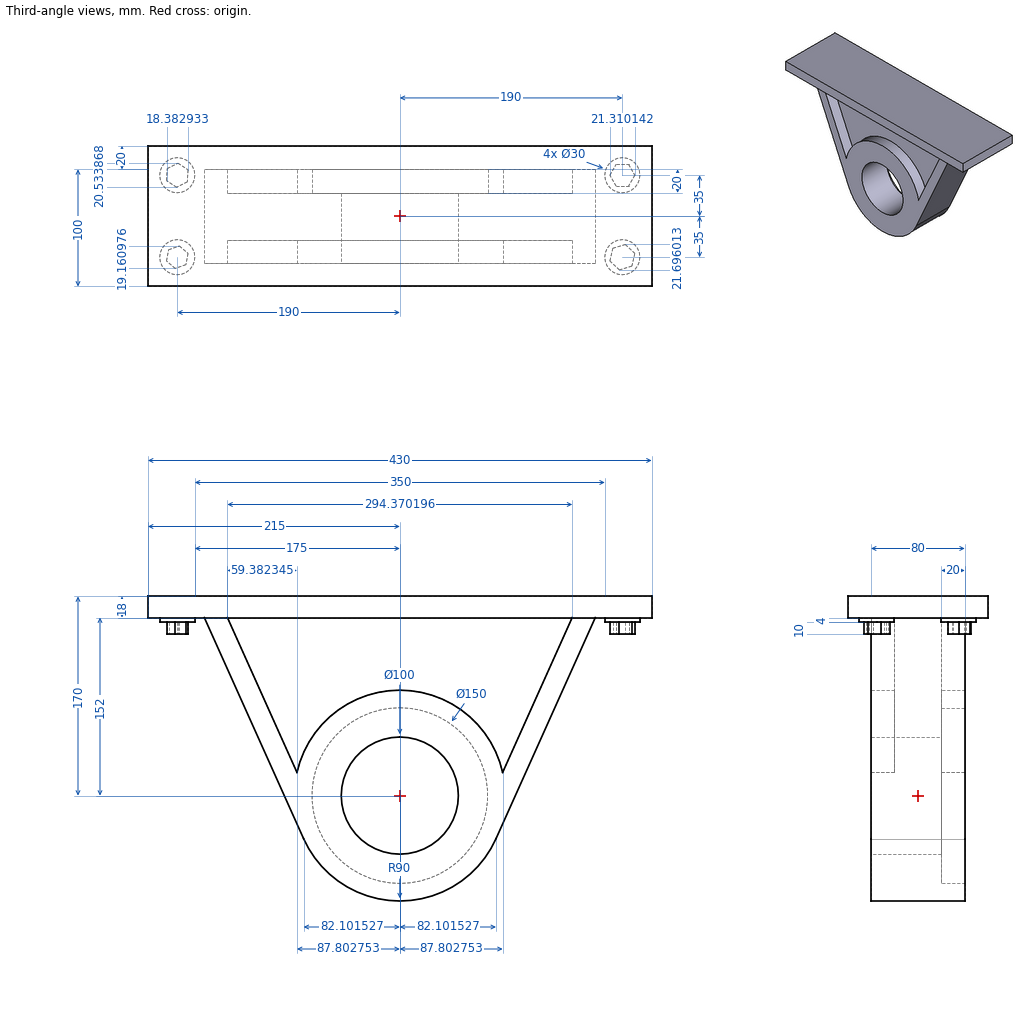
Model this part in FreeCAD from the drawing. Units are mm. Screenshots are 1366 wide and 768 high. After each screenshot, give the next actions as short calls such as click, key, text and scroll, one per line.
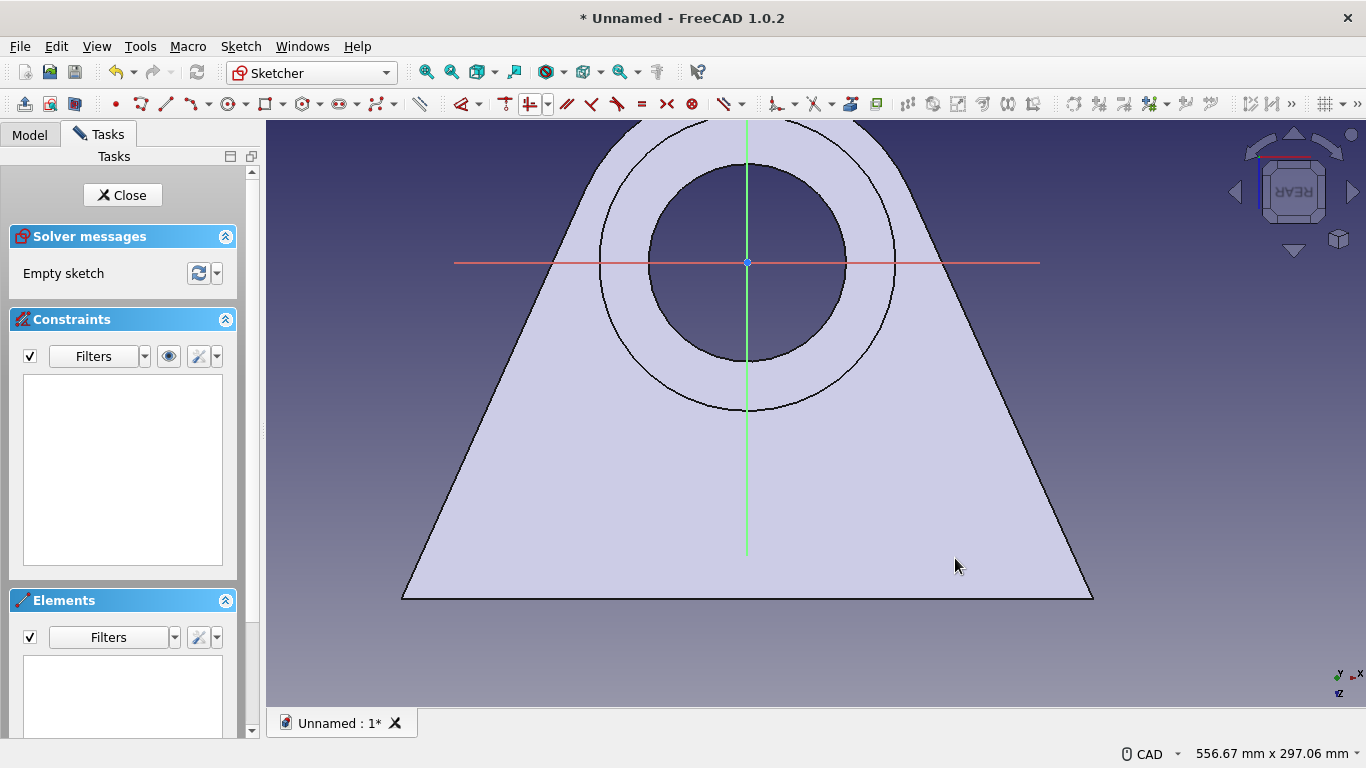
click(141, 104)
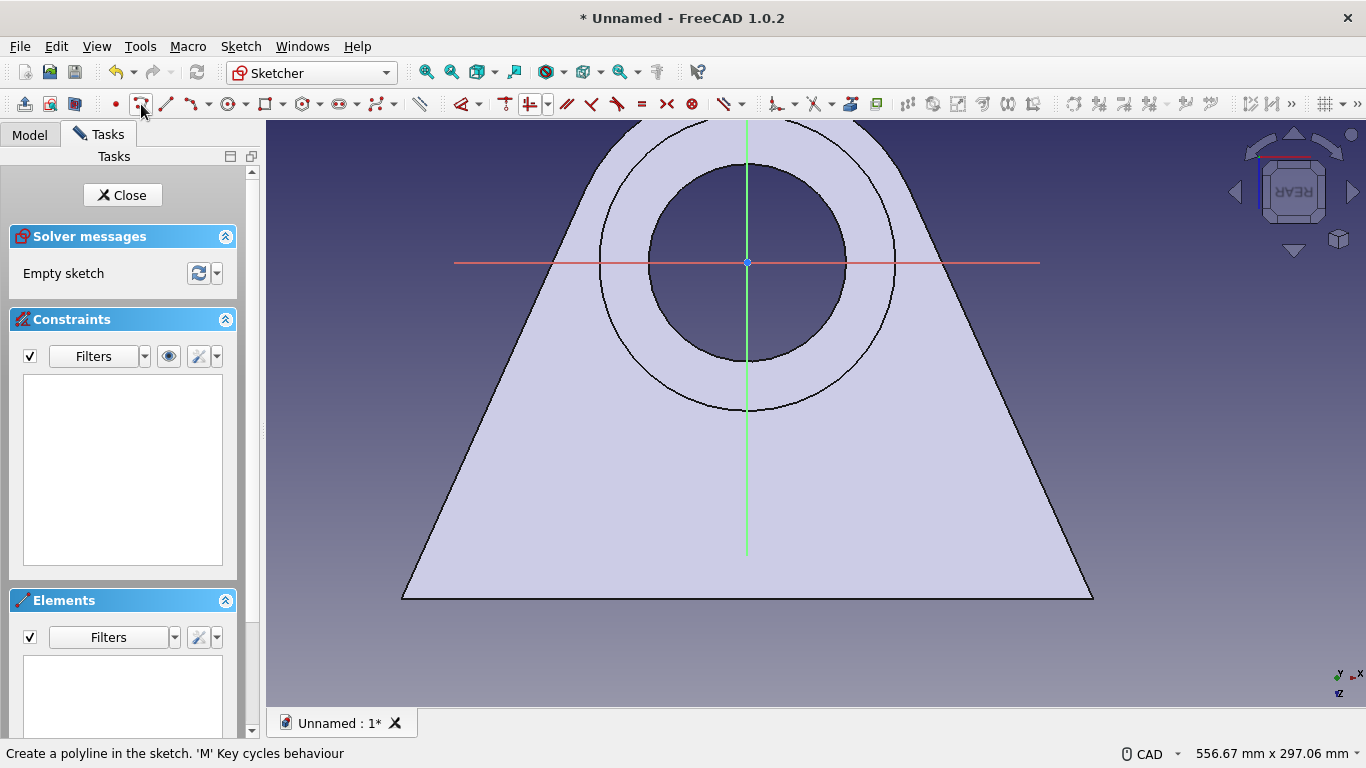
click(574, 302)
click(456, 563)
click(1038, 563)
click(921, 302)
right_click(921, 302)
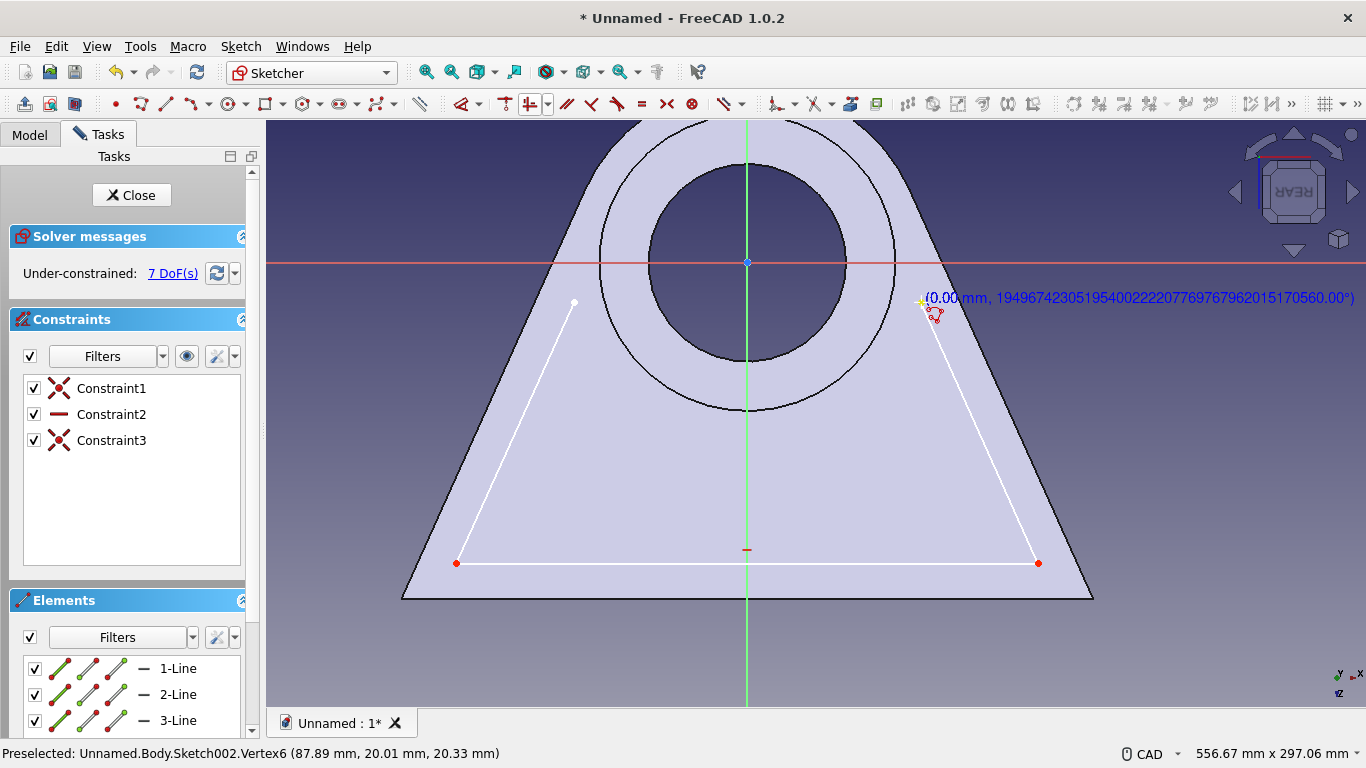
click(190, 104)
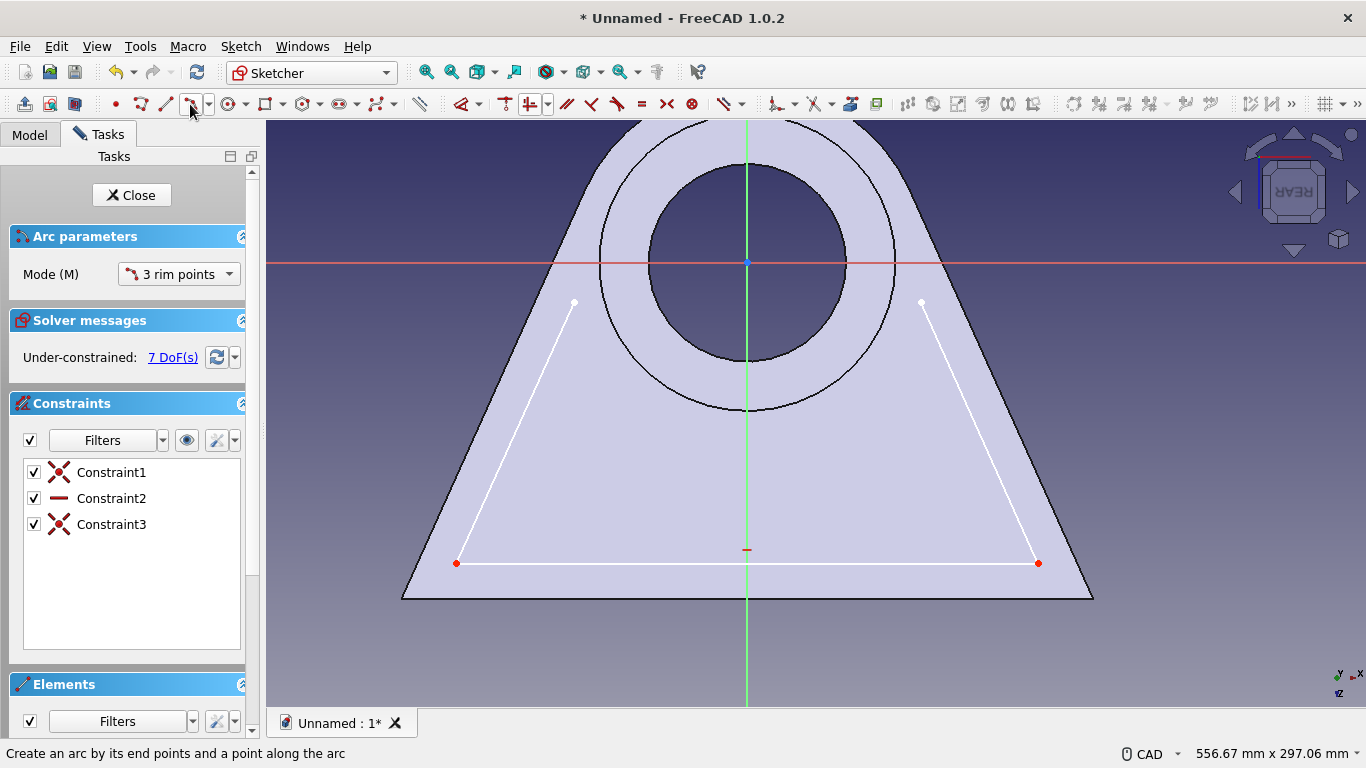
click(921, 303)
click(574, 303)
click(700, 434)
key(Escape)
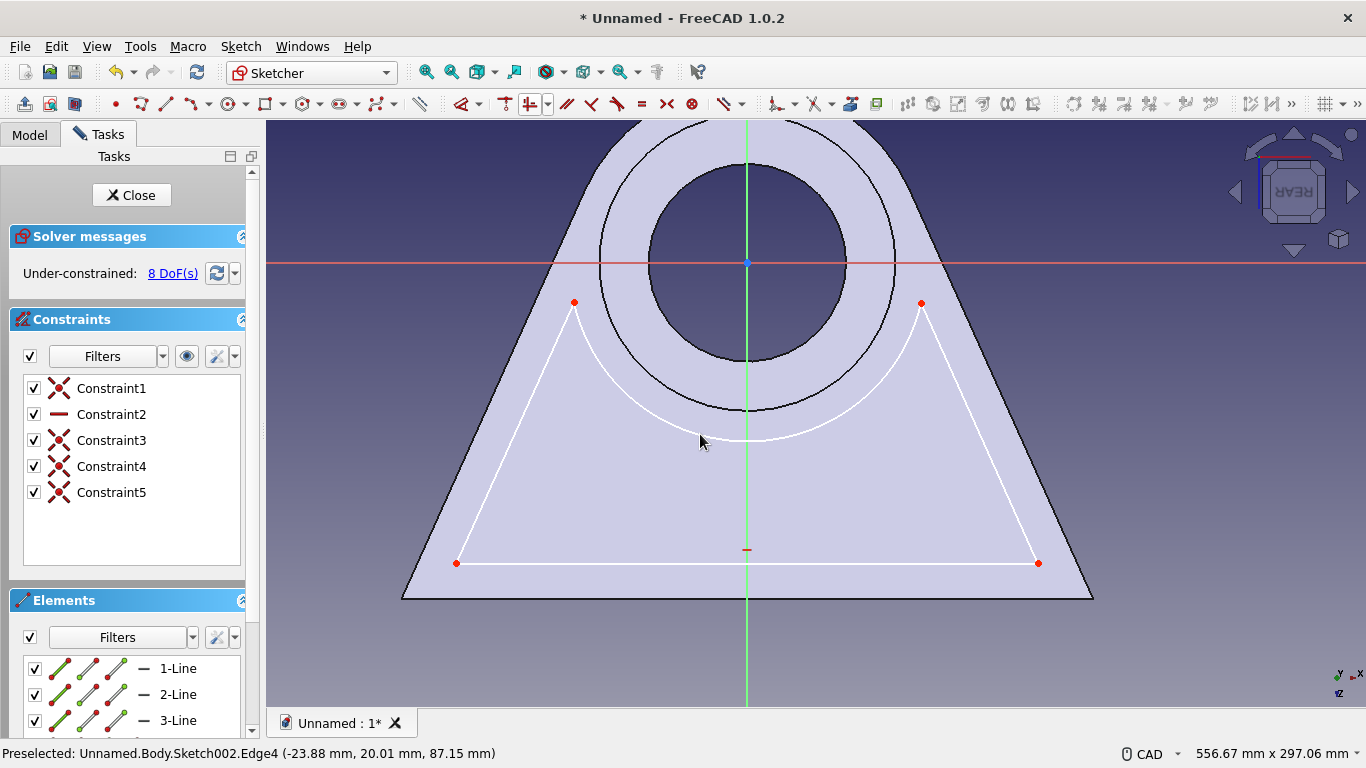
drag(737, 253, 758, 274)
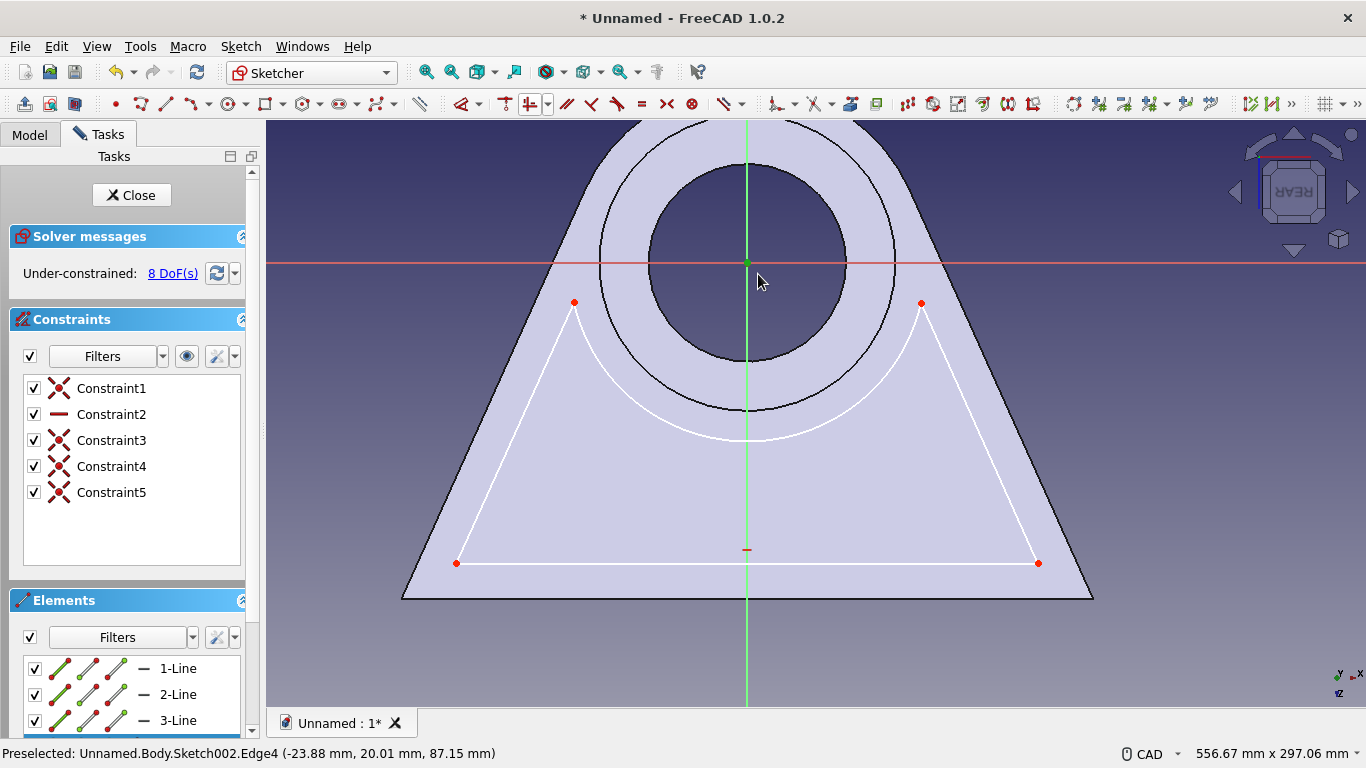
click(505, 104)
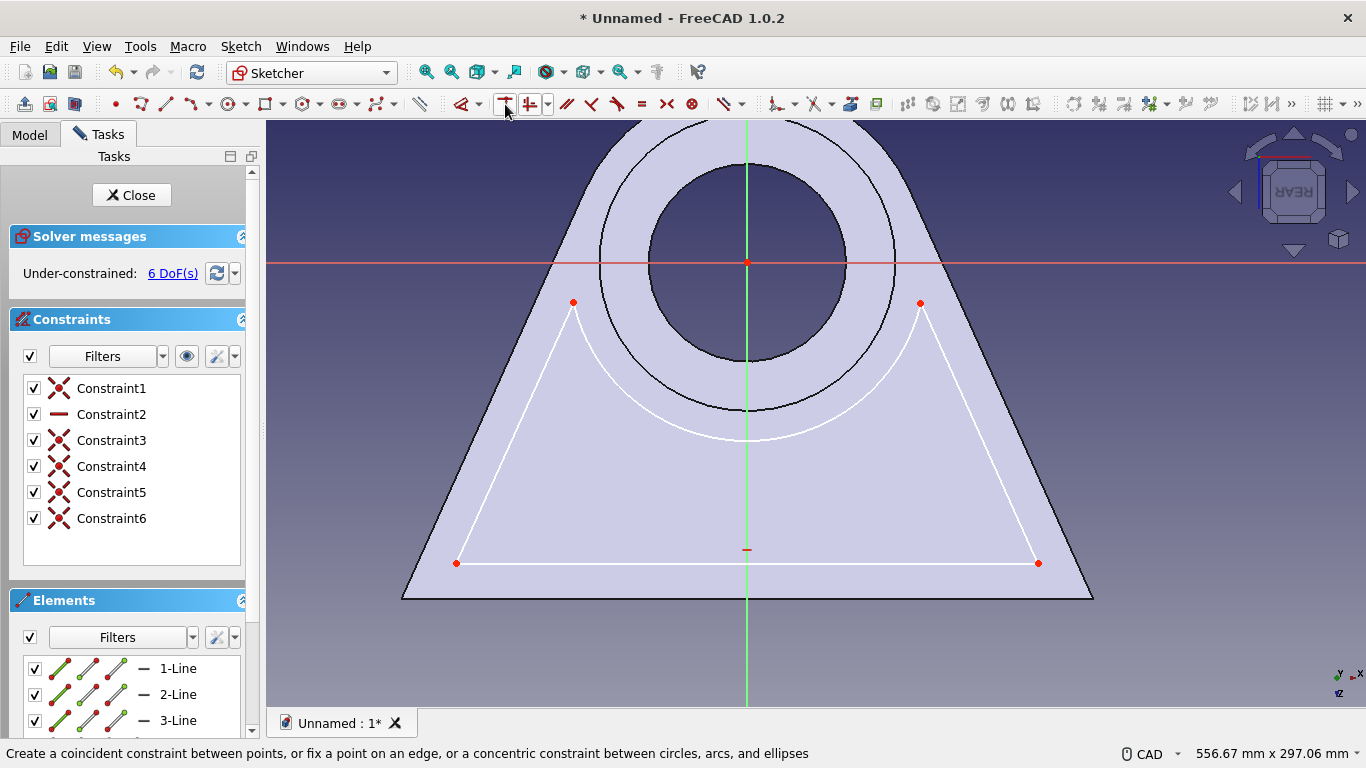
click(460, 104)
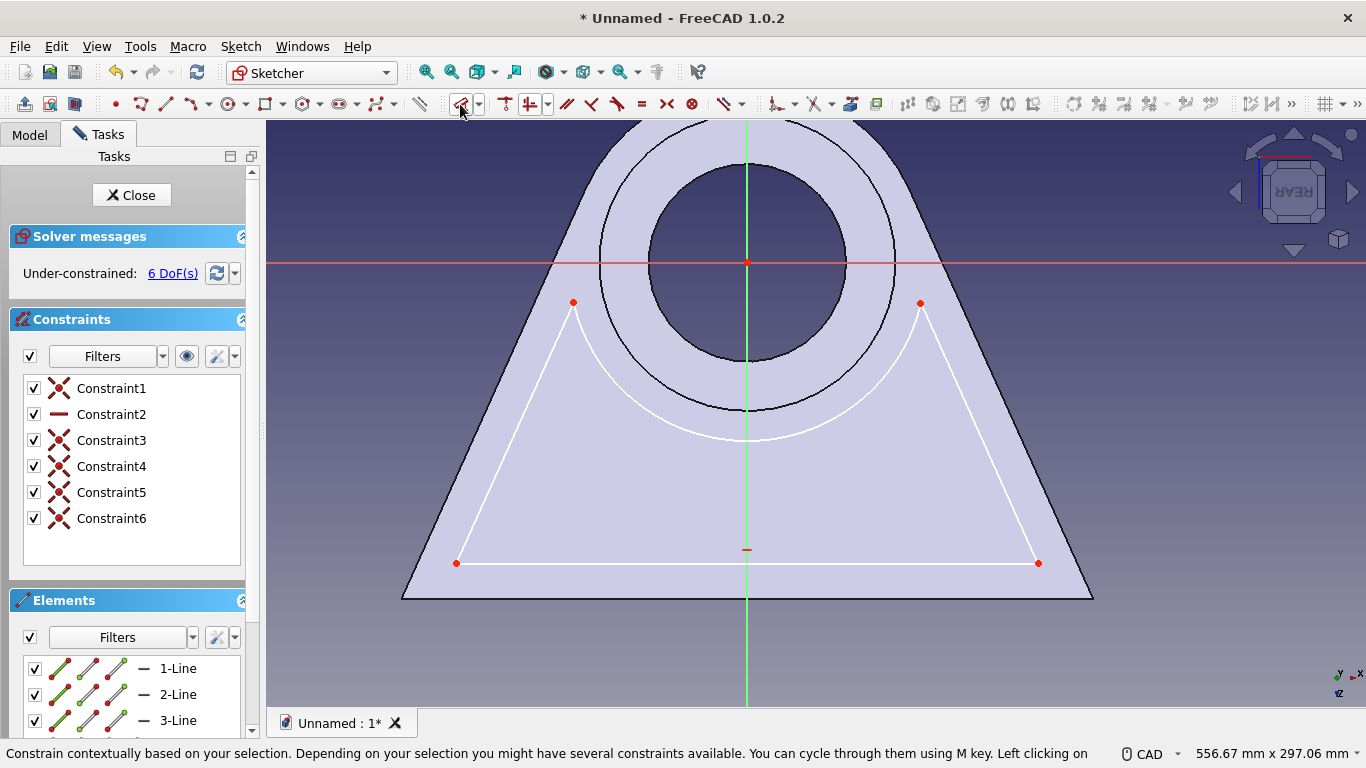
click(656, 416)
click(640, 443)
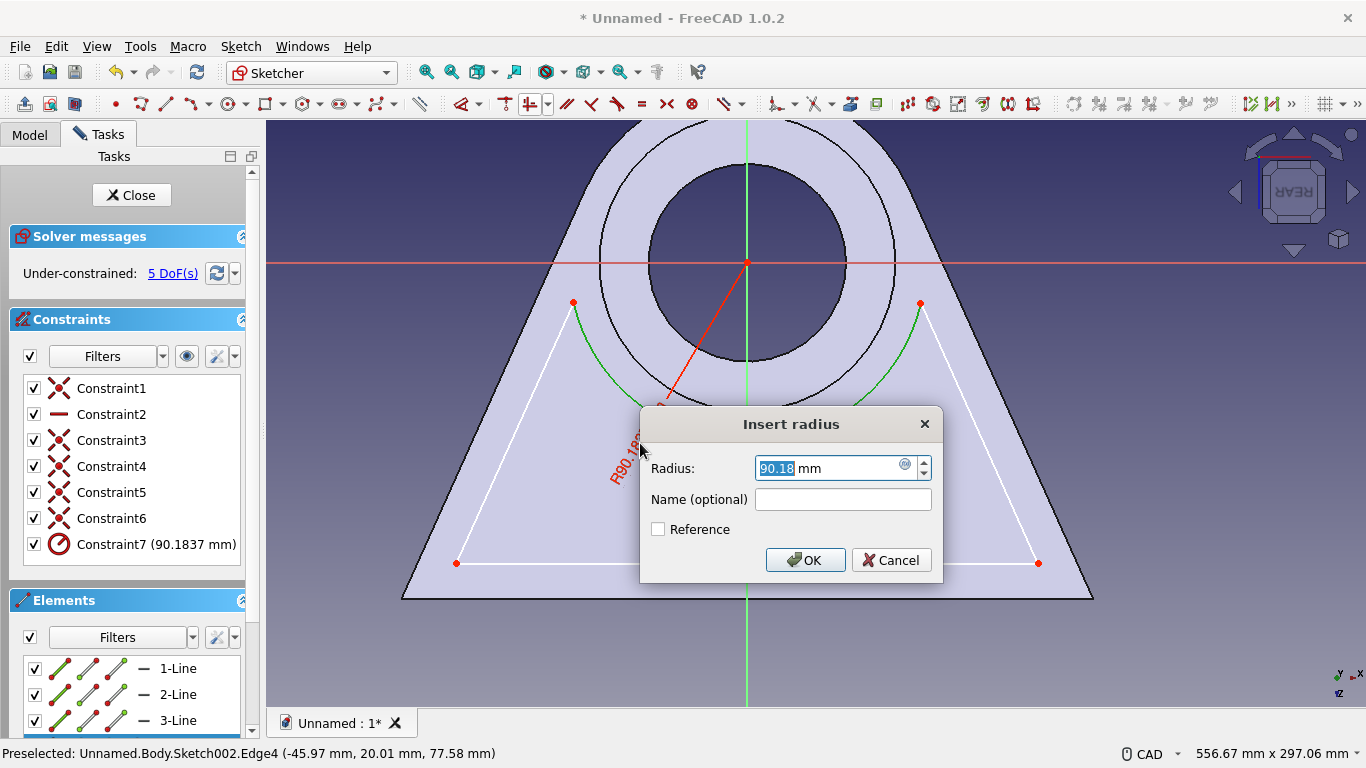
text(90)
key(Return)